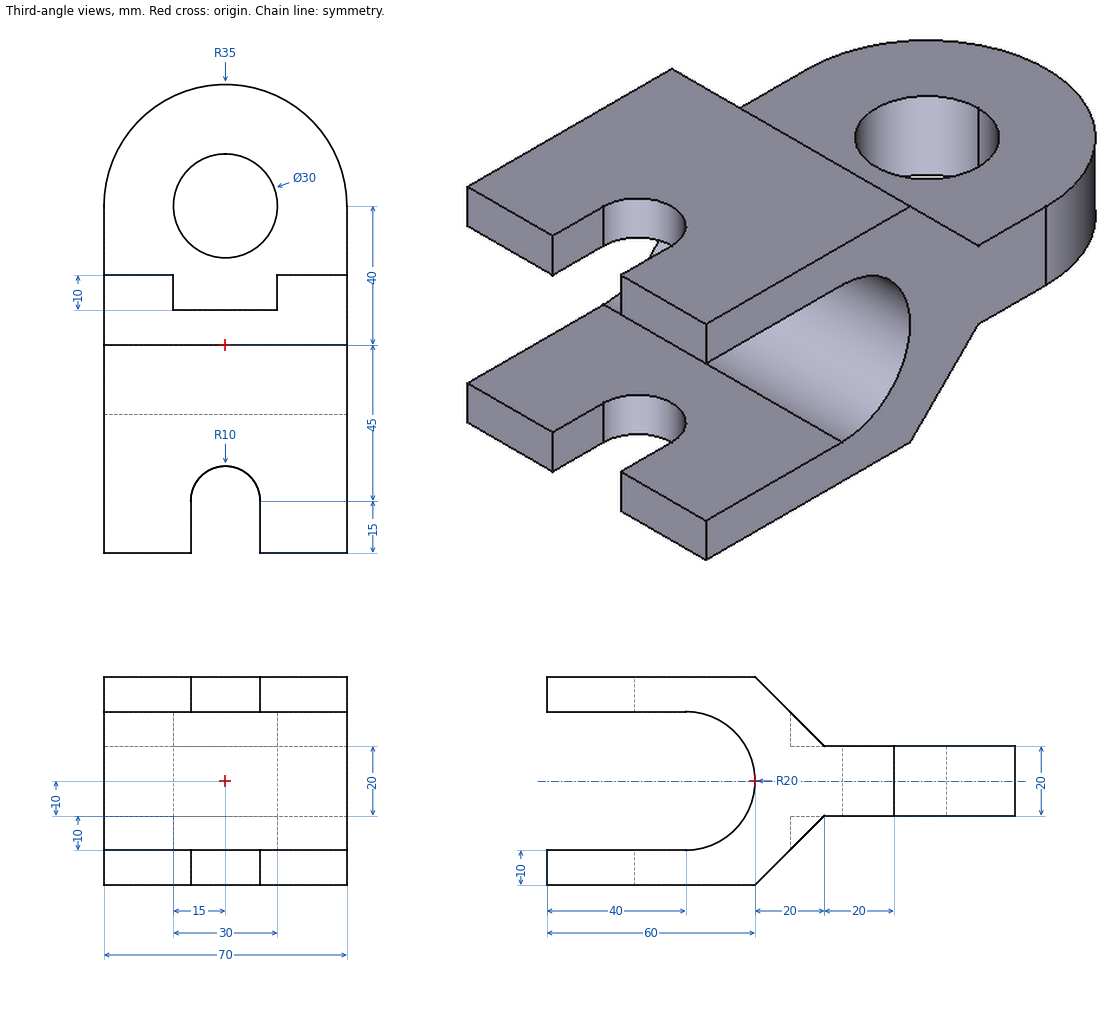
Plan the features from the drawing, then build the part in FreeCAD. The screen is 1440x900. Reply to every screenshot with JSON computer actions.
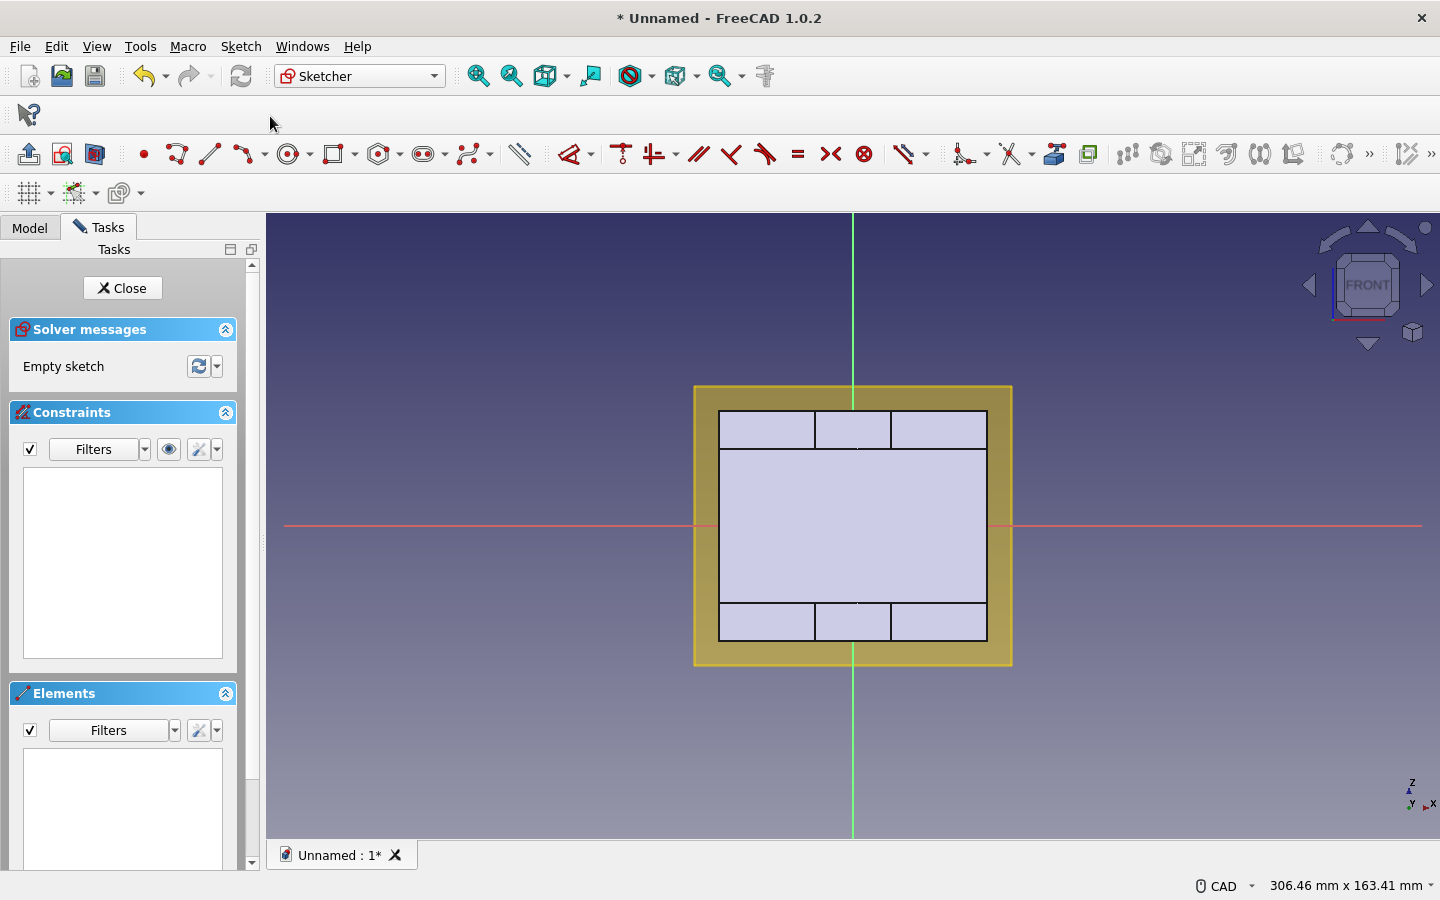
{"action": "left_click", "coordinate": [95, 154]}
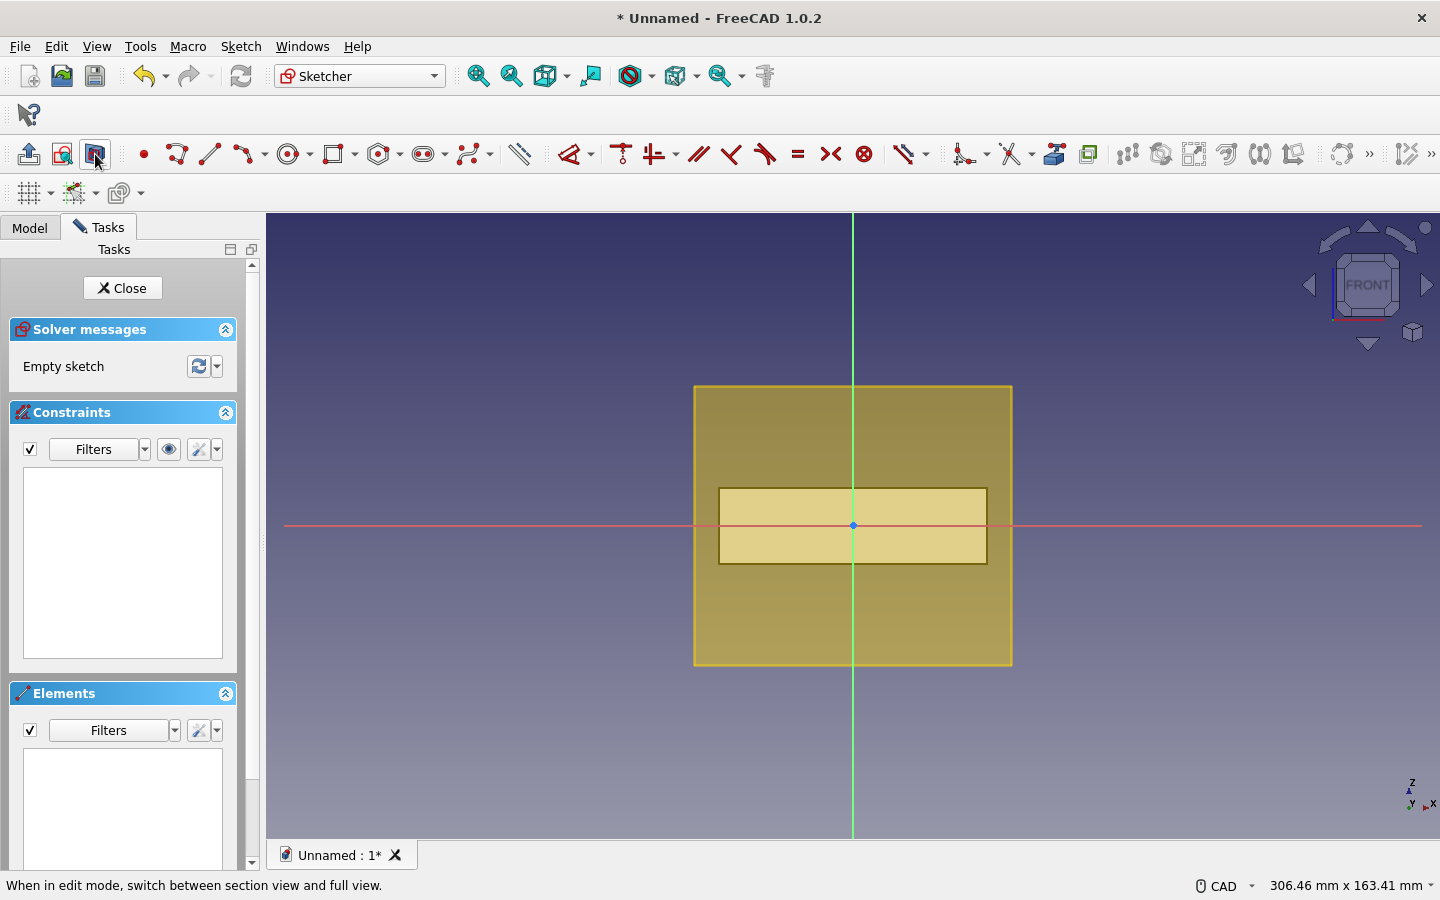
{"action": "scroll", "coordinate": [870, 574], "scroll_direction": "up", "scroll_amount": 8}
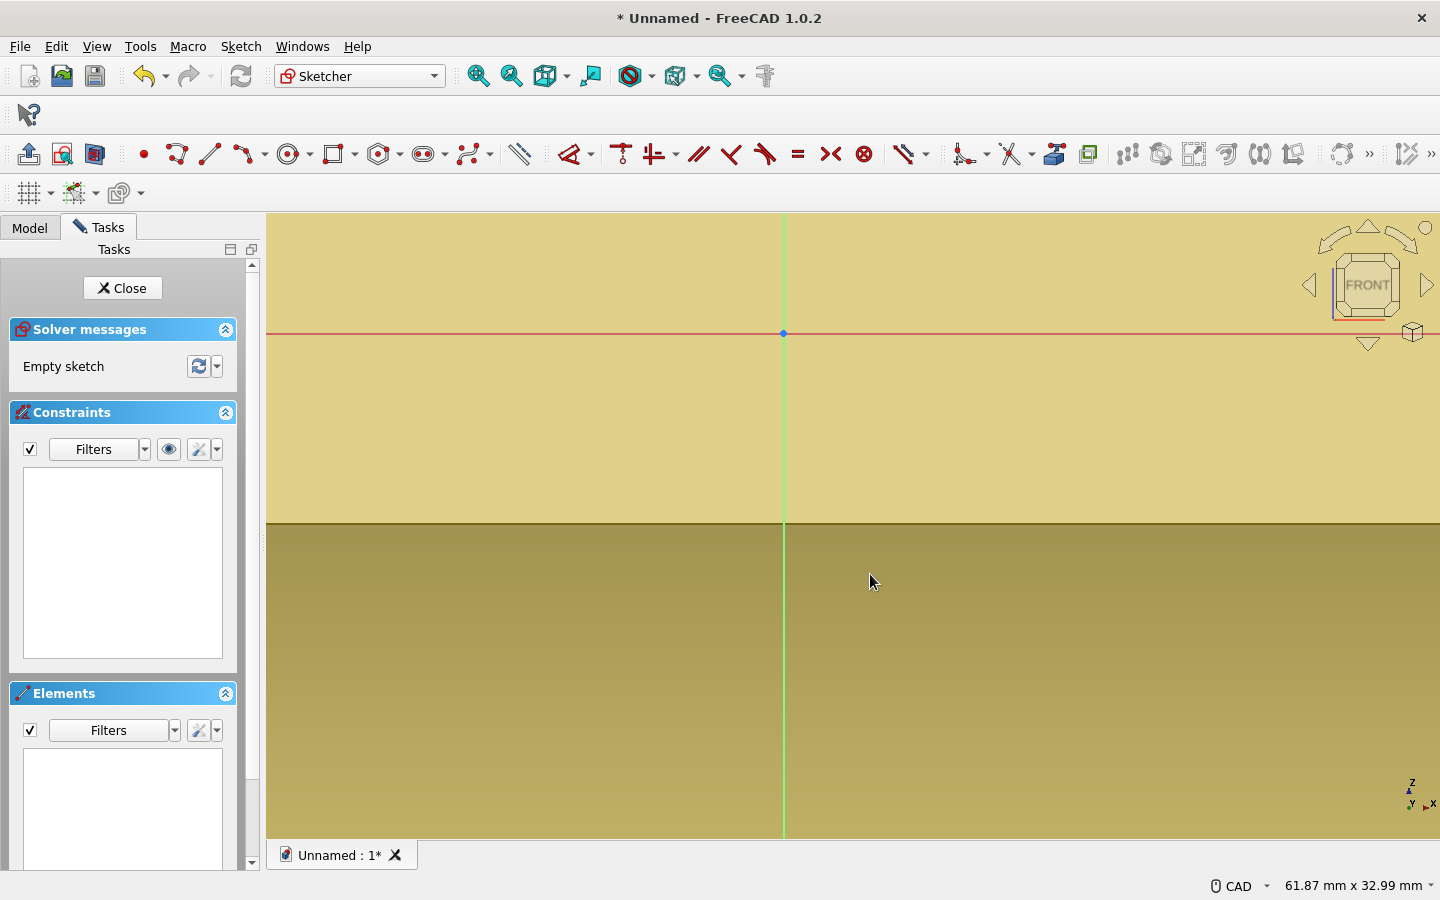
{"action": "key", "text": "g r"}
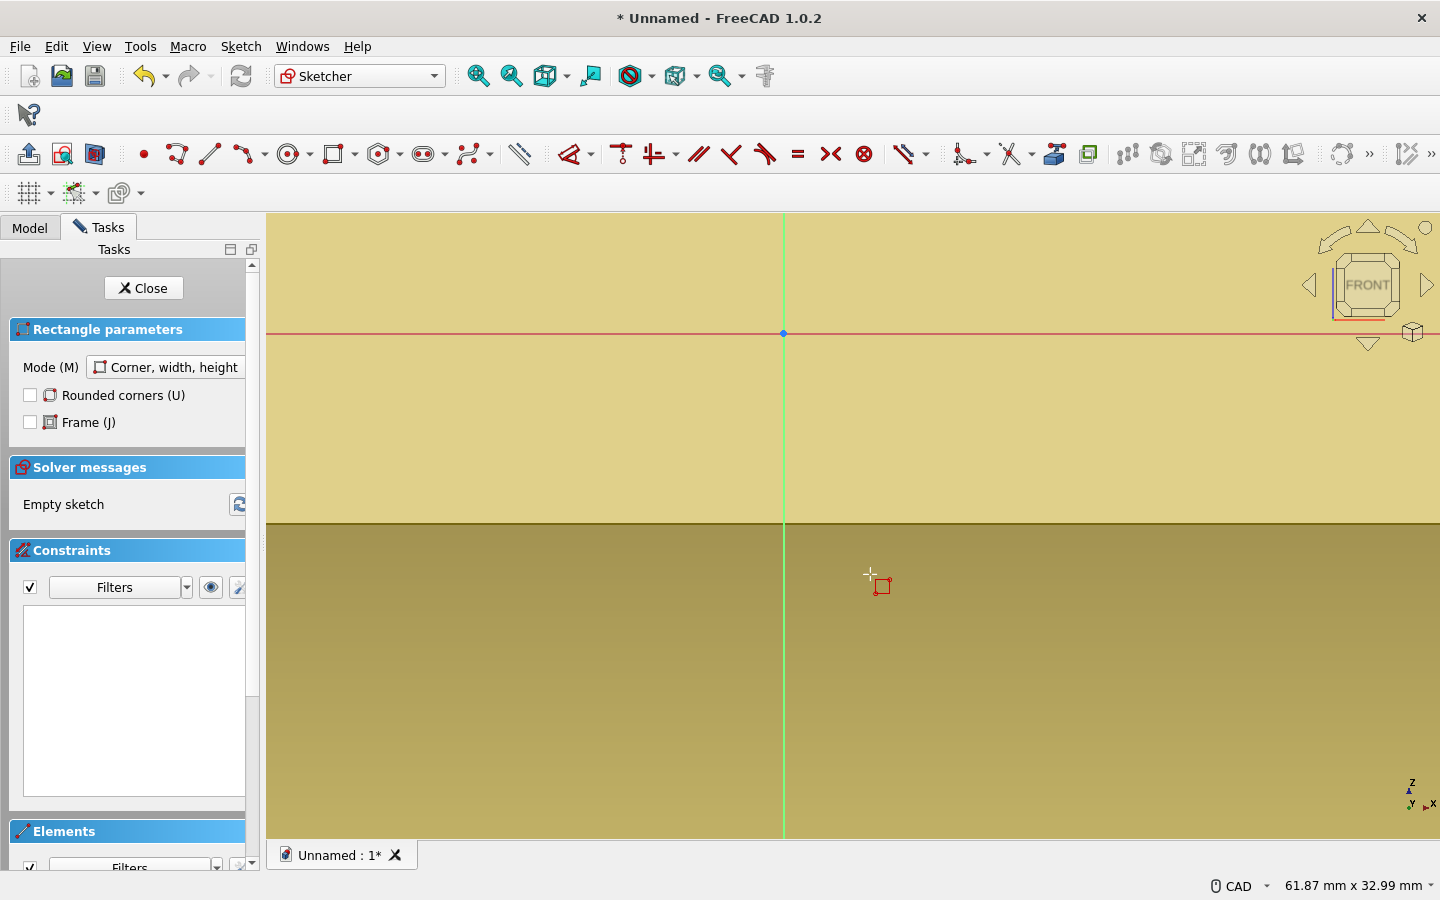
{"action": "left_click", "coordinate": [499, 524]}
{"action": "left_click", "coordinate": [1068, 713]}
{"action": "key", "text": "Escape"}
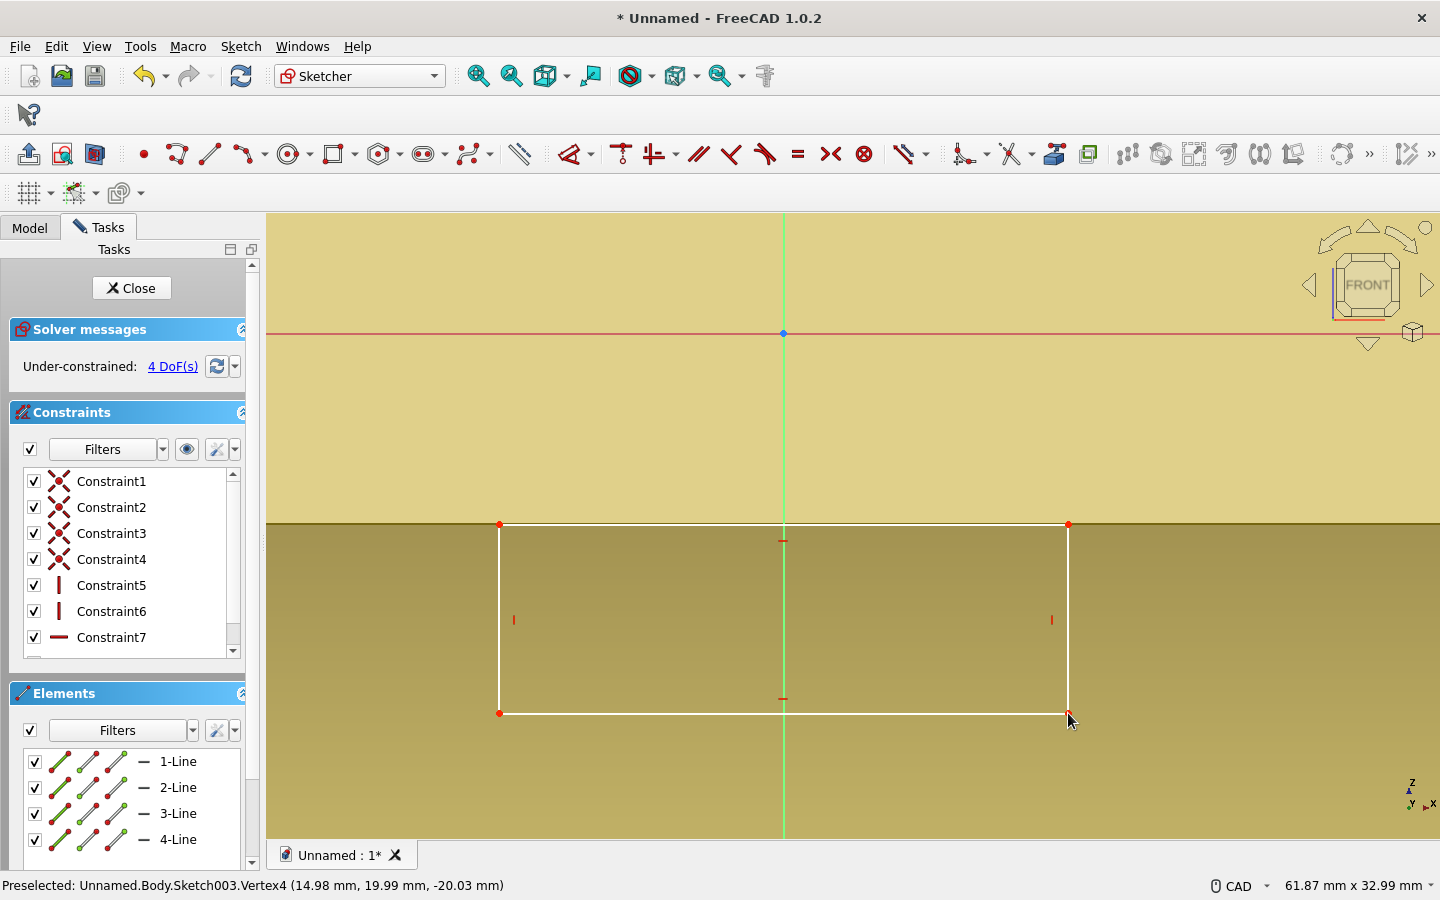
{"action": "left_click", "coordinate": [568, 154]}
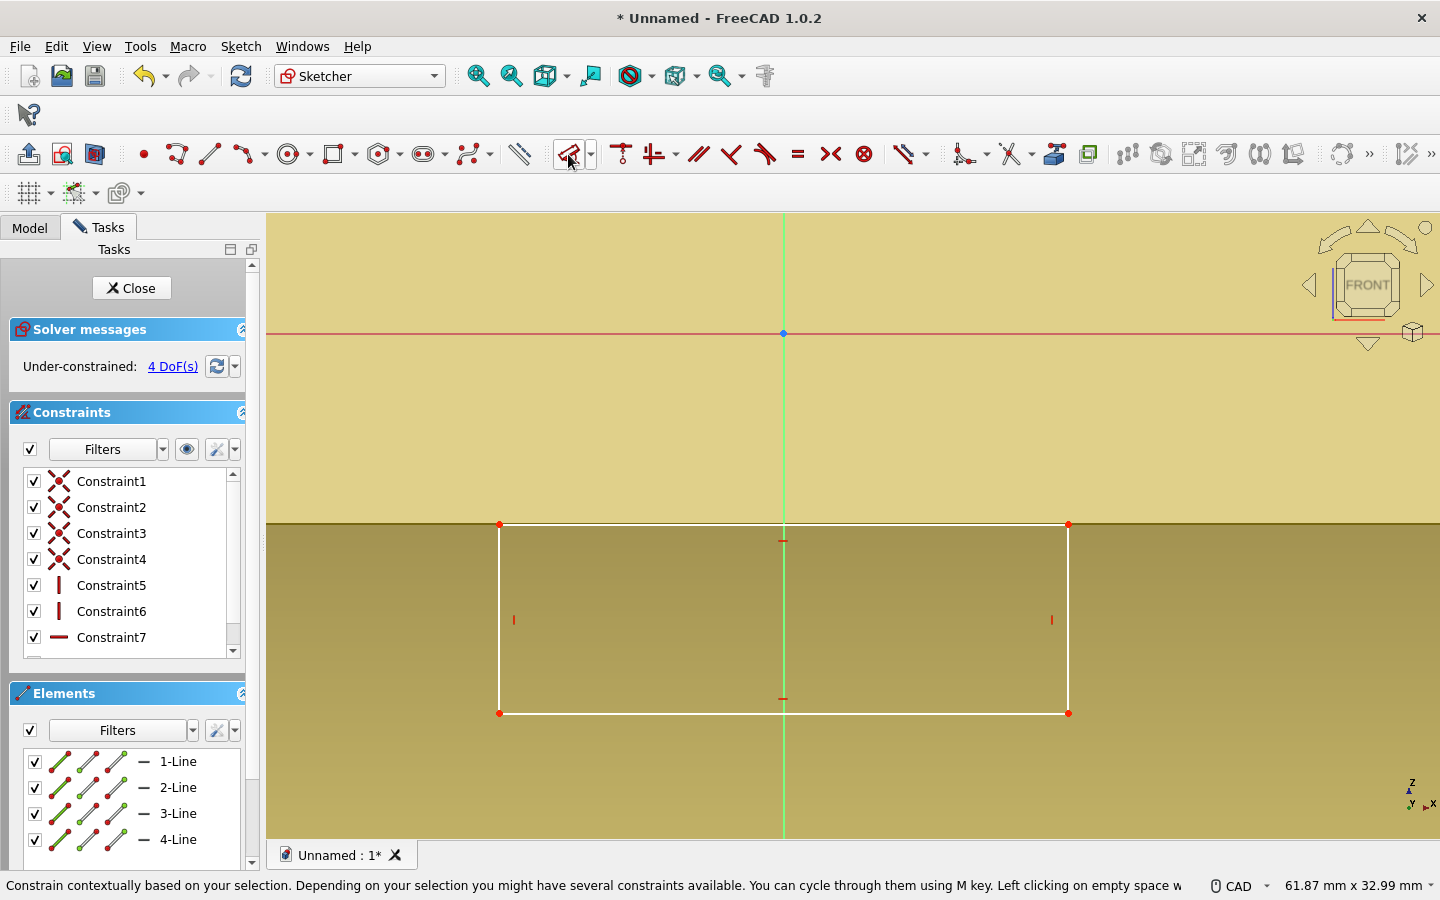
{"action": "left_click", "coordinate": [499, 582]}
{"action": "left_click", "coordinate": [465, 619]}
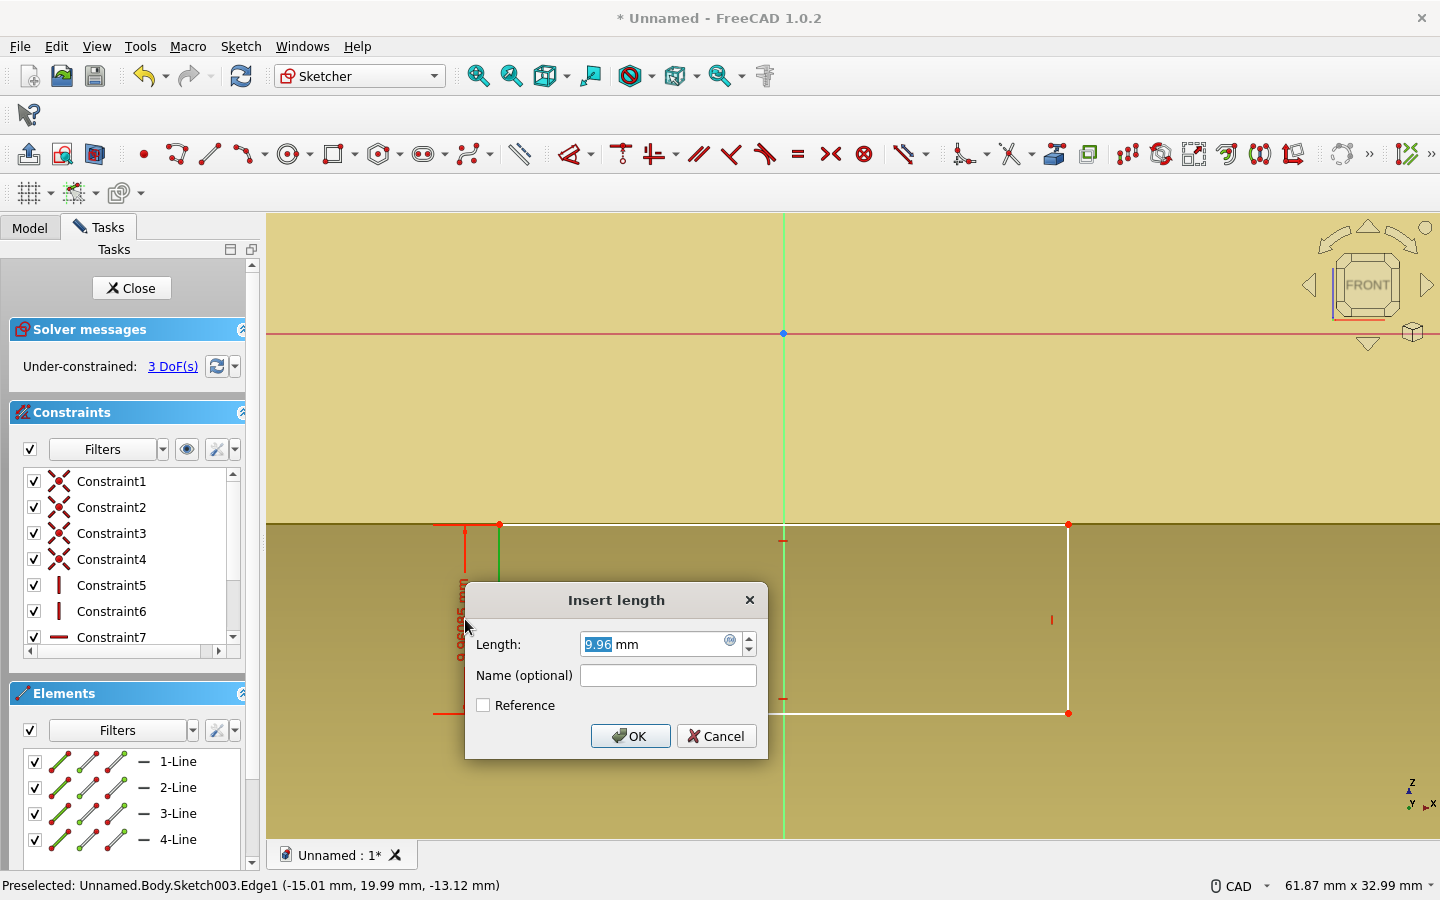
{"action": "type", "text": "10"}
{"action": "key", "text": "Return"}